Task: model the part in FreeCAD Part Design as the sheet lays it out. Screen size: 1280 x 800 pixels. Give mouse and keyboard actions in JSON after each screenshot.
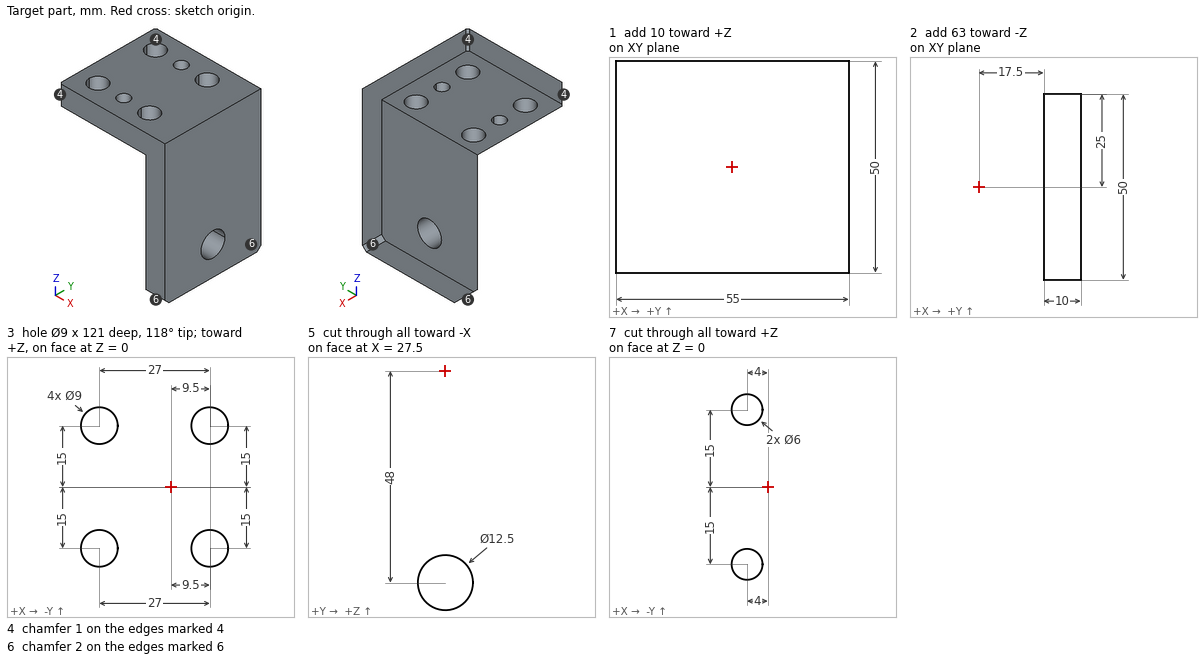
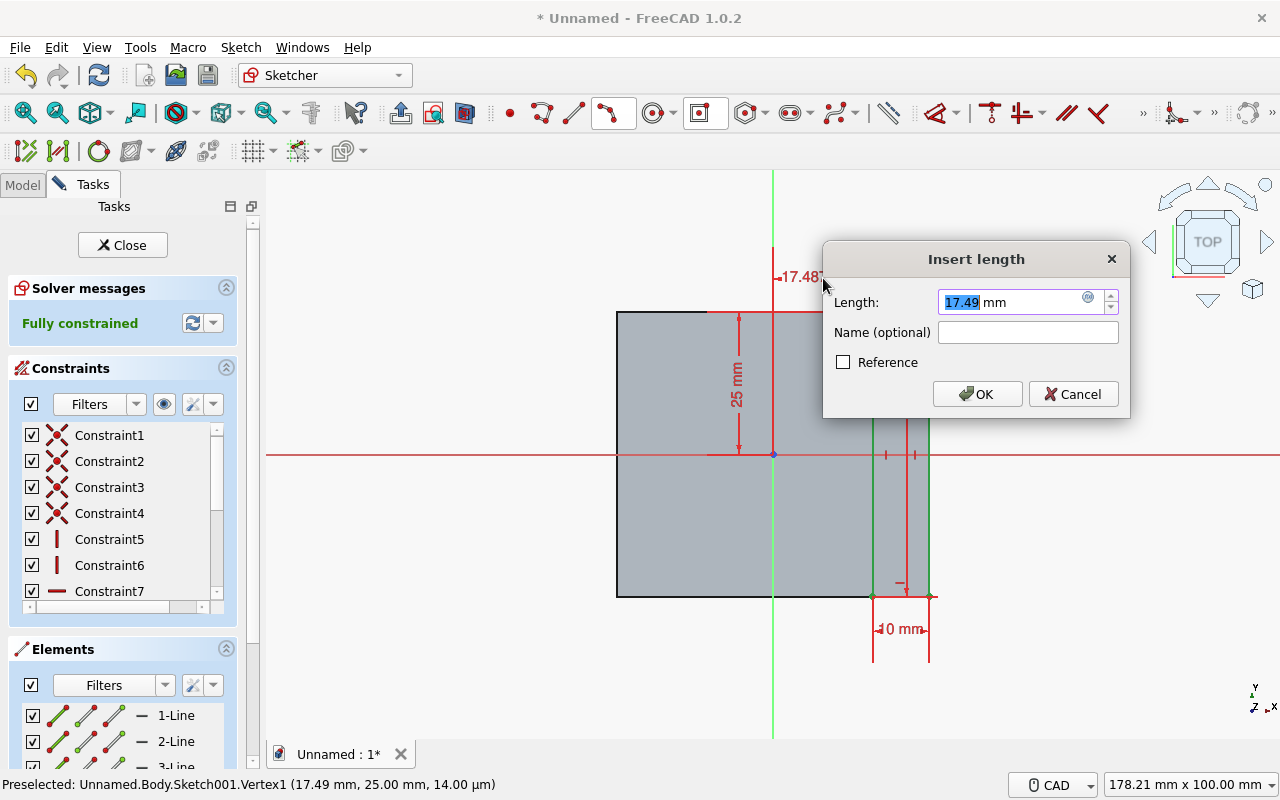
{"action": "type", "text": "17.5"}
{"action": "key", "text": "Return"}
{"action": "key", "text": "Escape"}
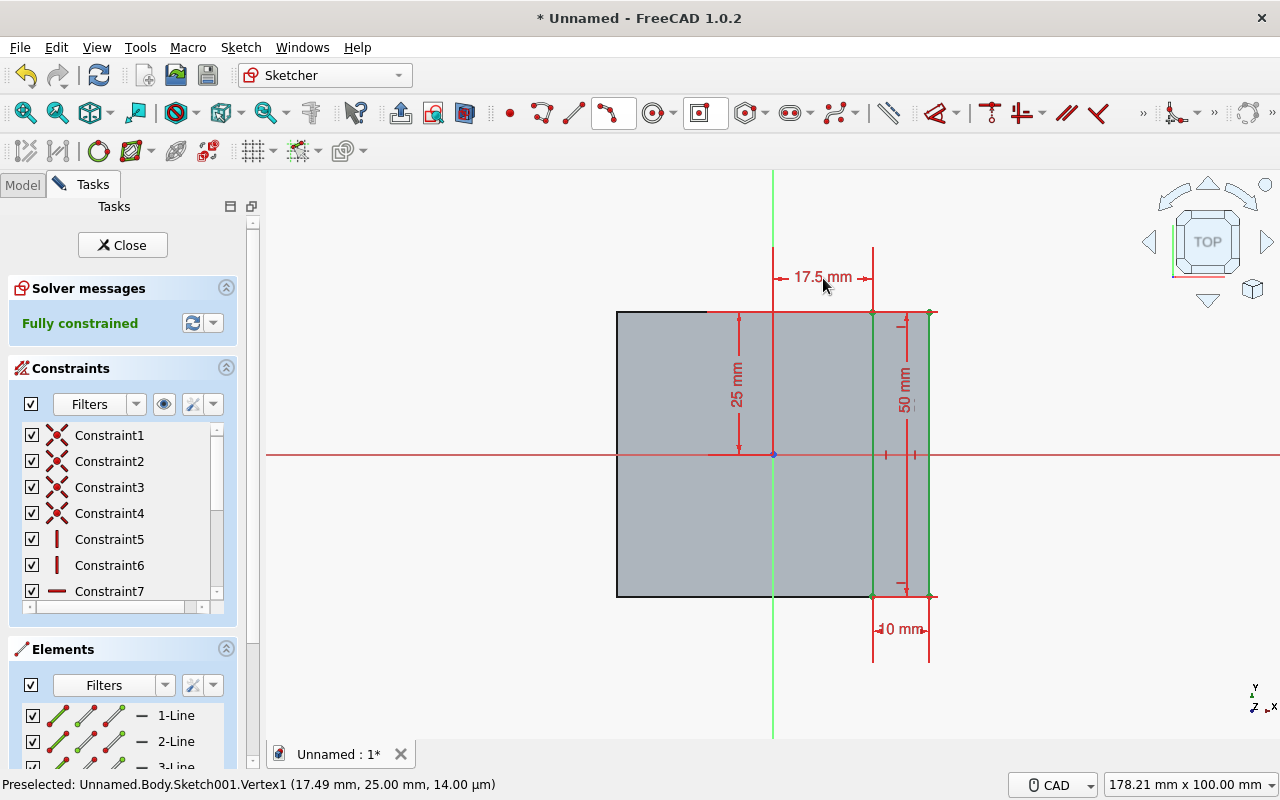
{"action": "left_click", "coordinate": [123, 245]}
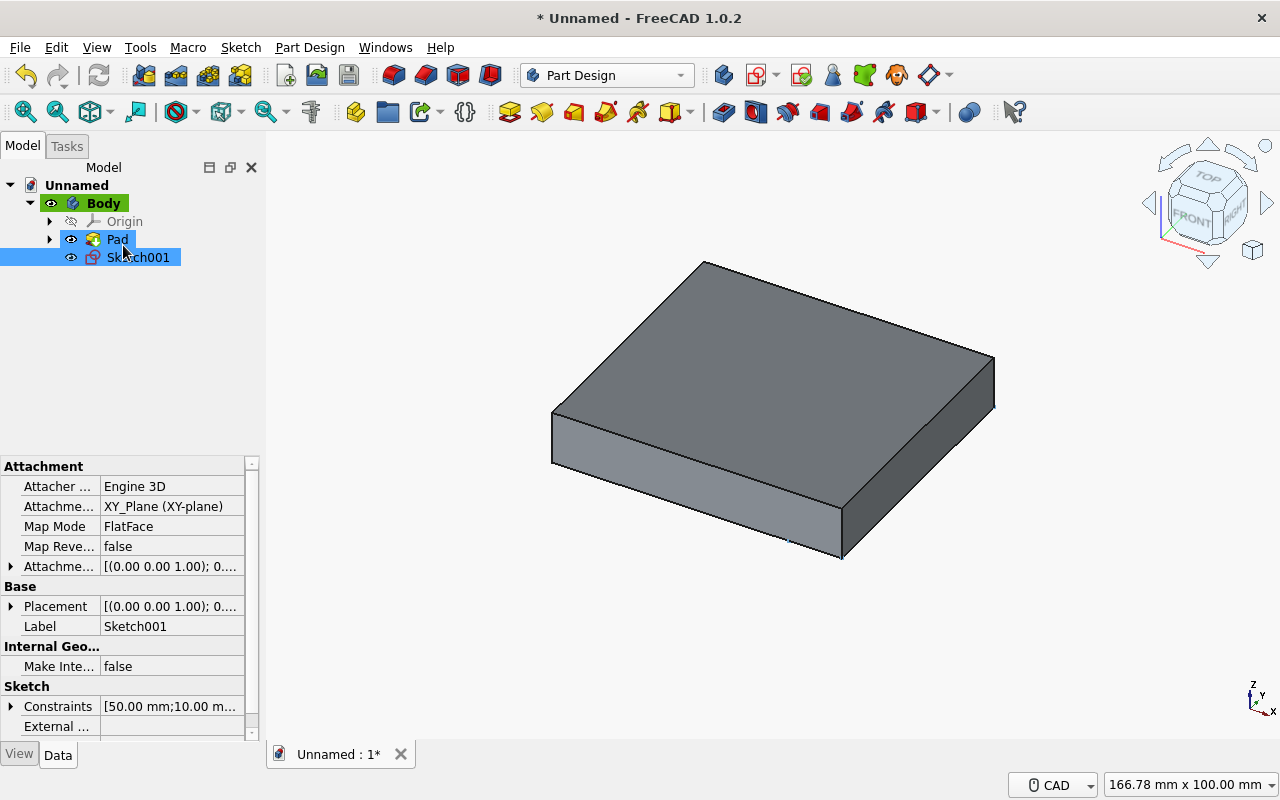
{"action": "left_click", "coordinate": [510, 112]}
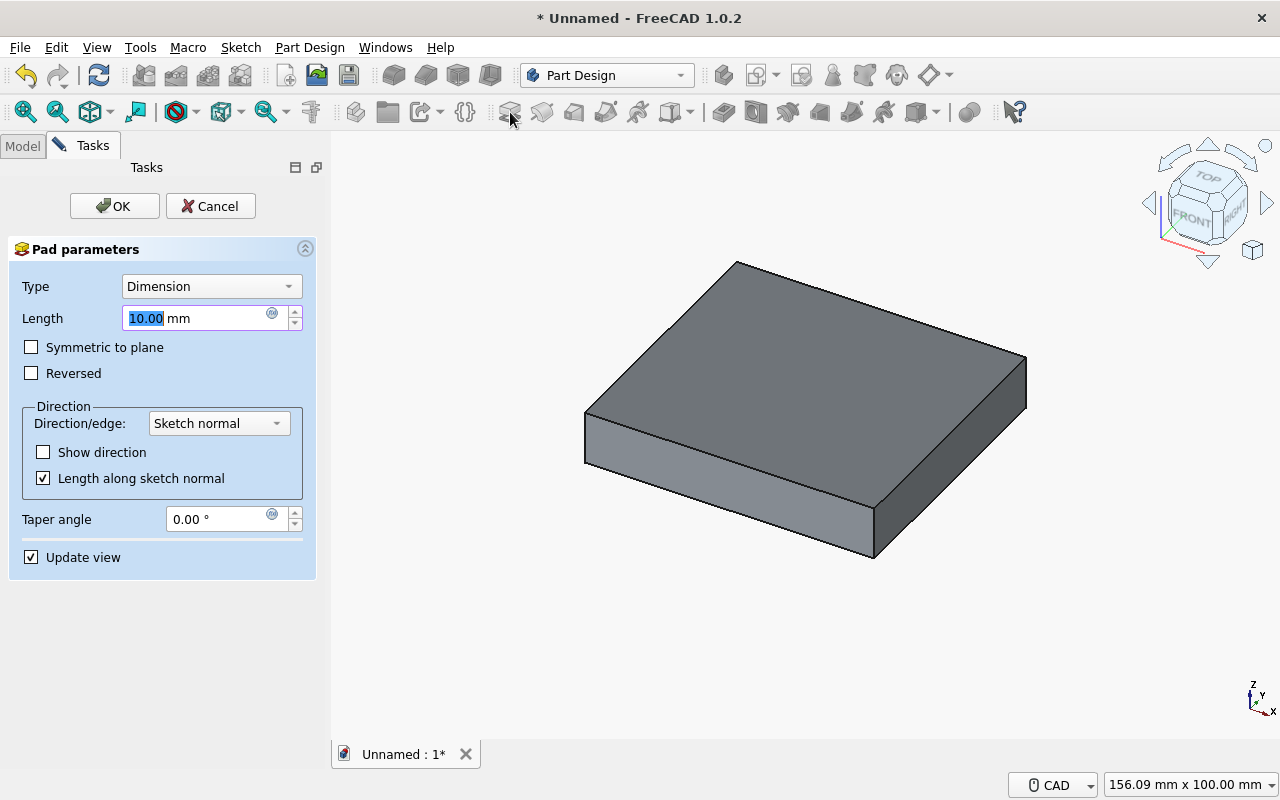
{"action": "type", "text": "63"}
{"action": "key", "text": "Tab"}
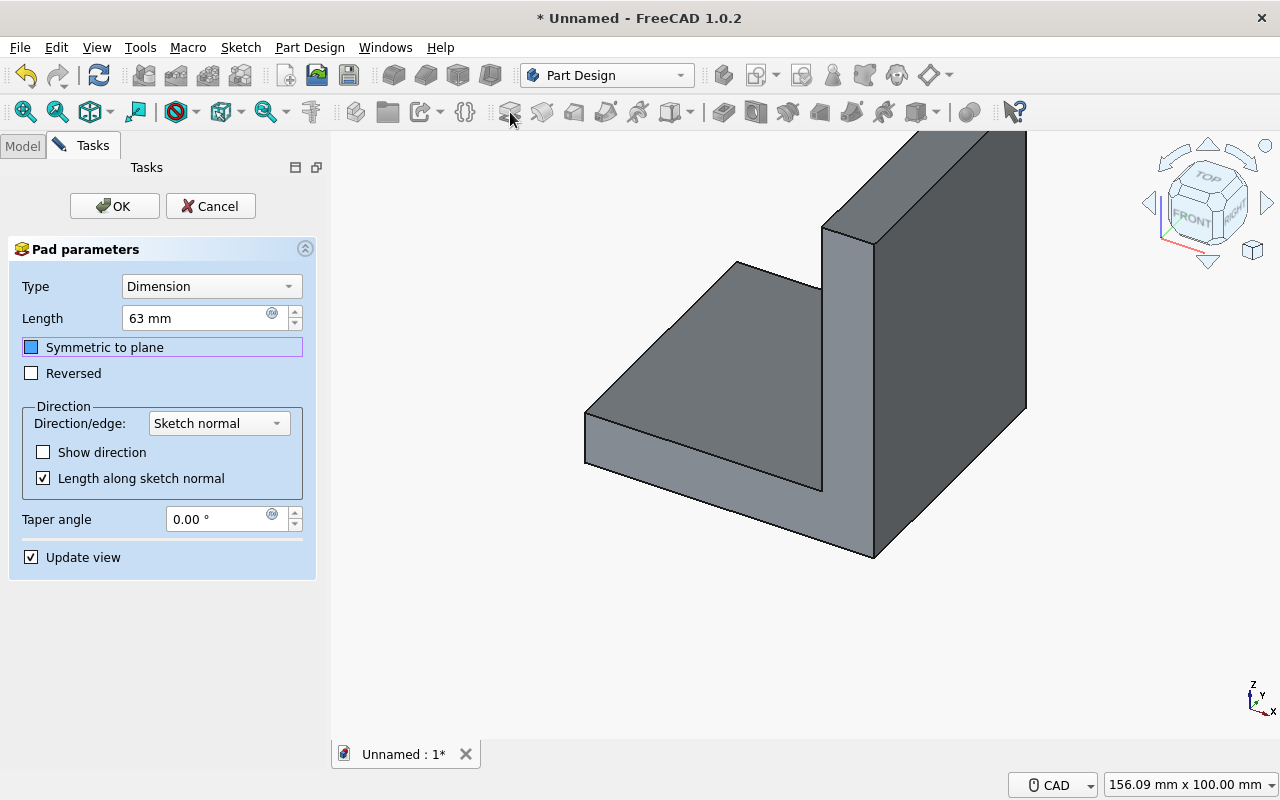
{"action": "left_click", "coordinate": [30, 373]}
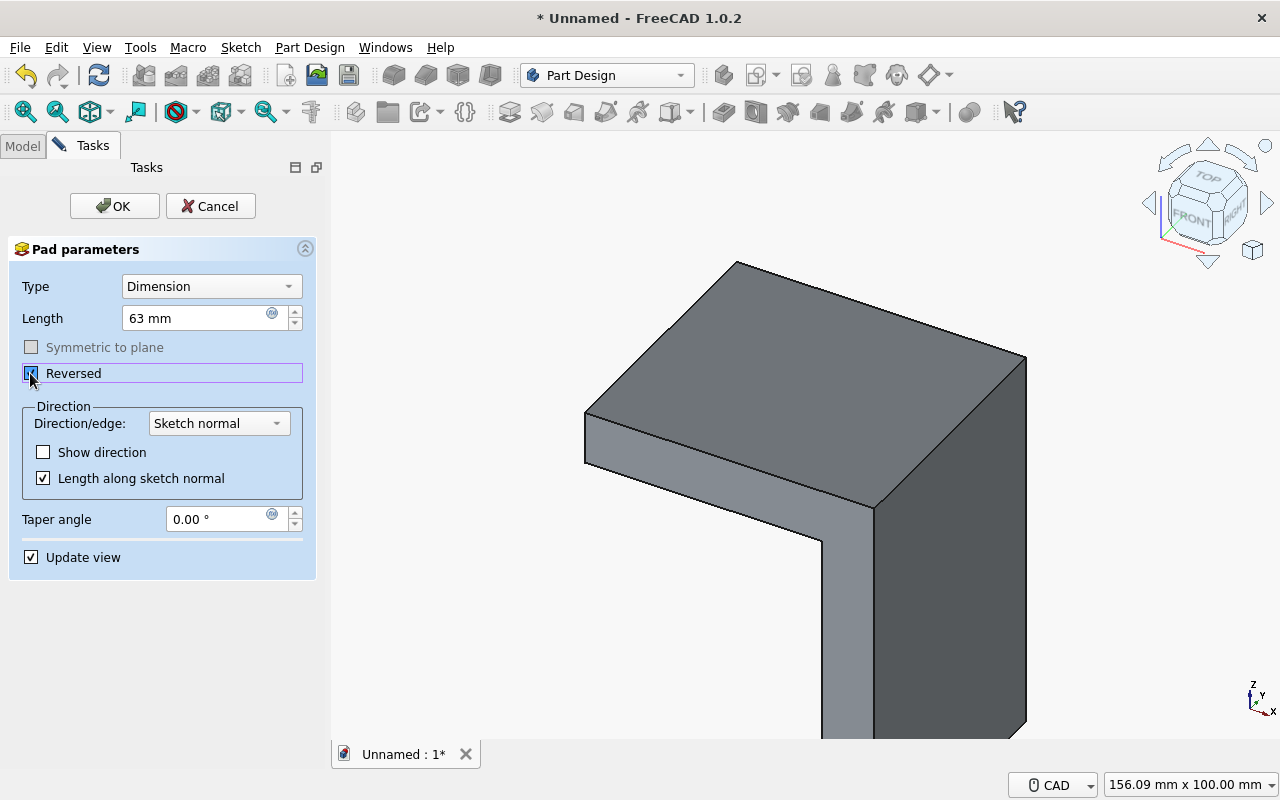
{"action": "left_click", "coordinate": [115, 206]}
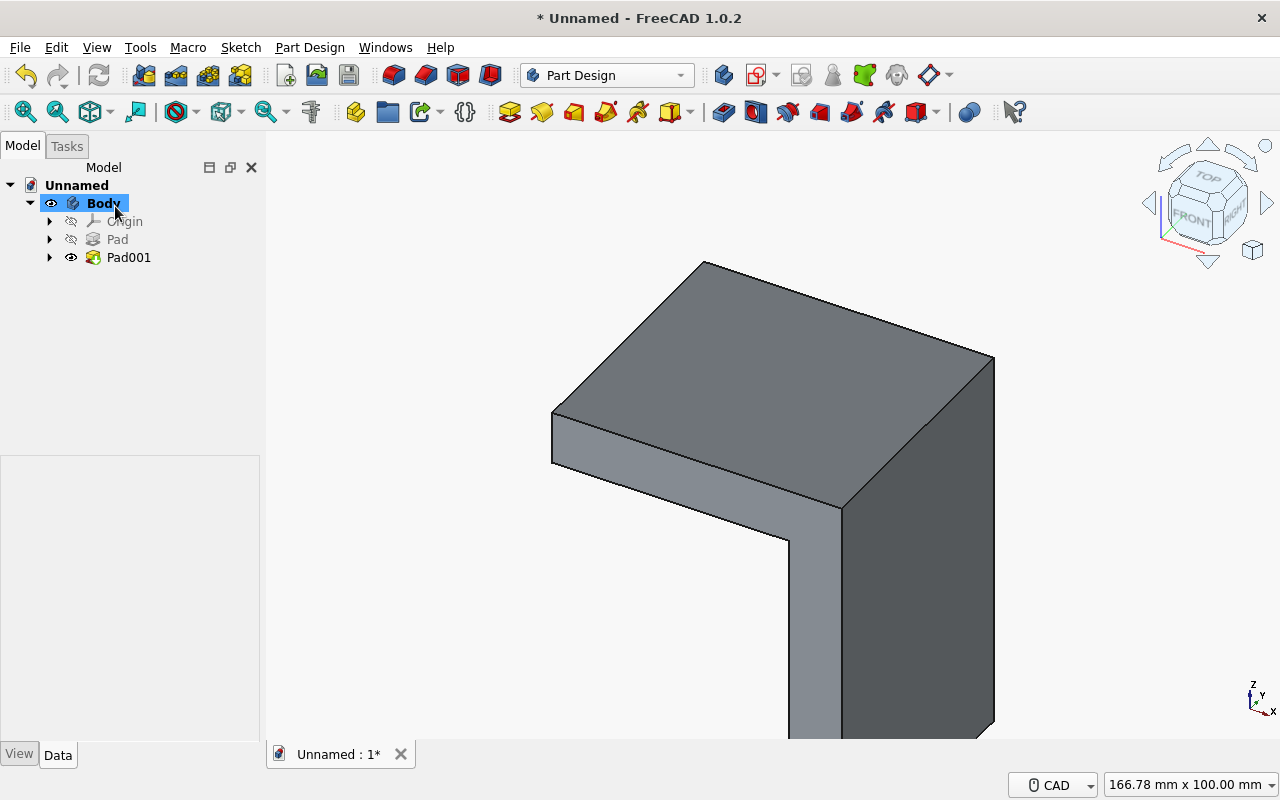
{"action": "key", "text": "v f"}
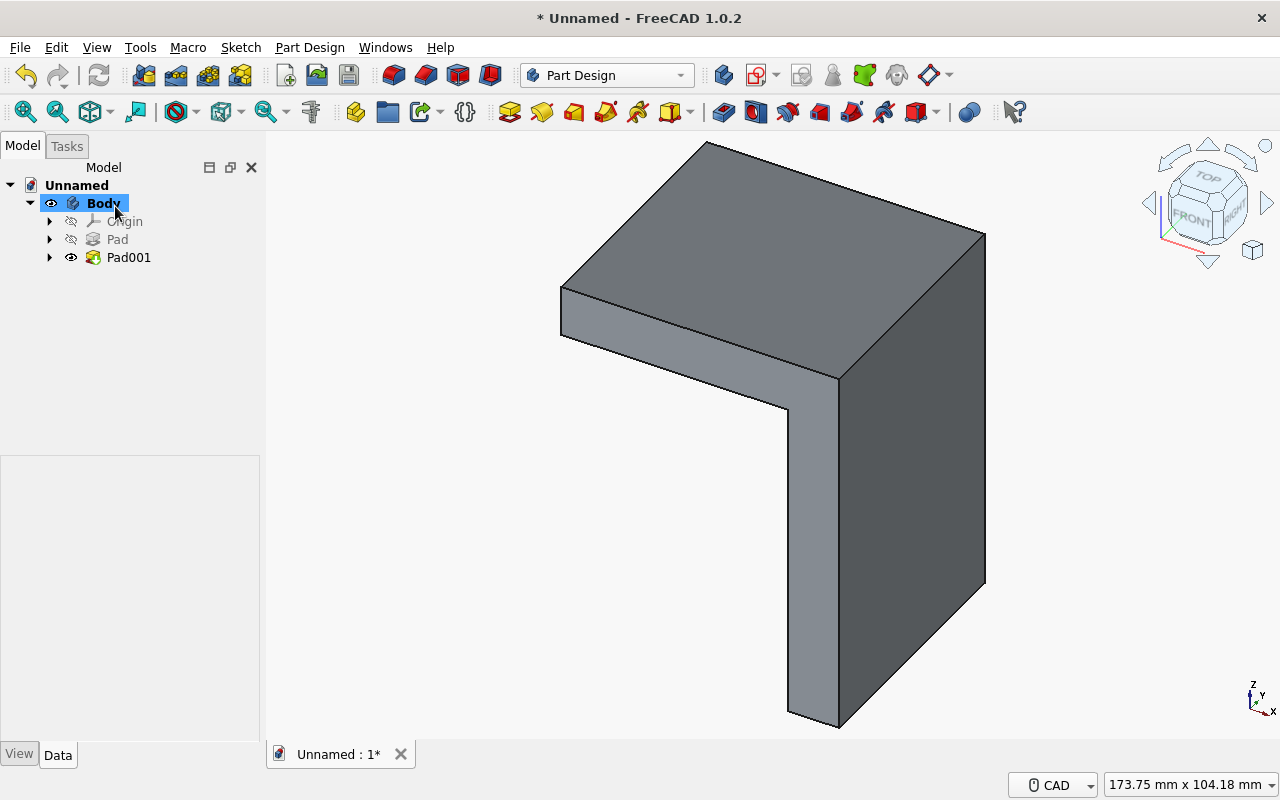
{"action": "key", "text": "5"}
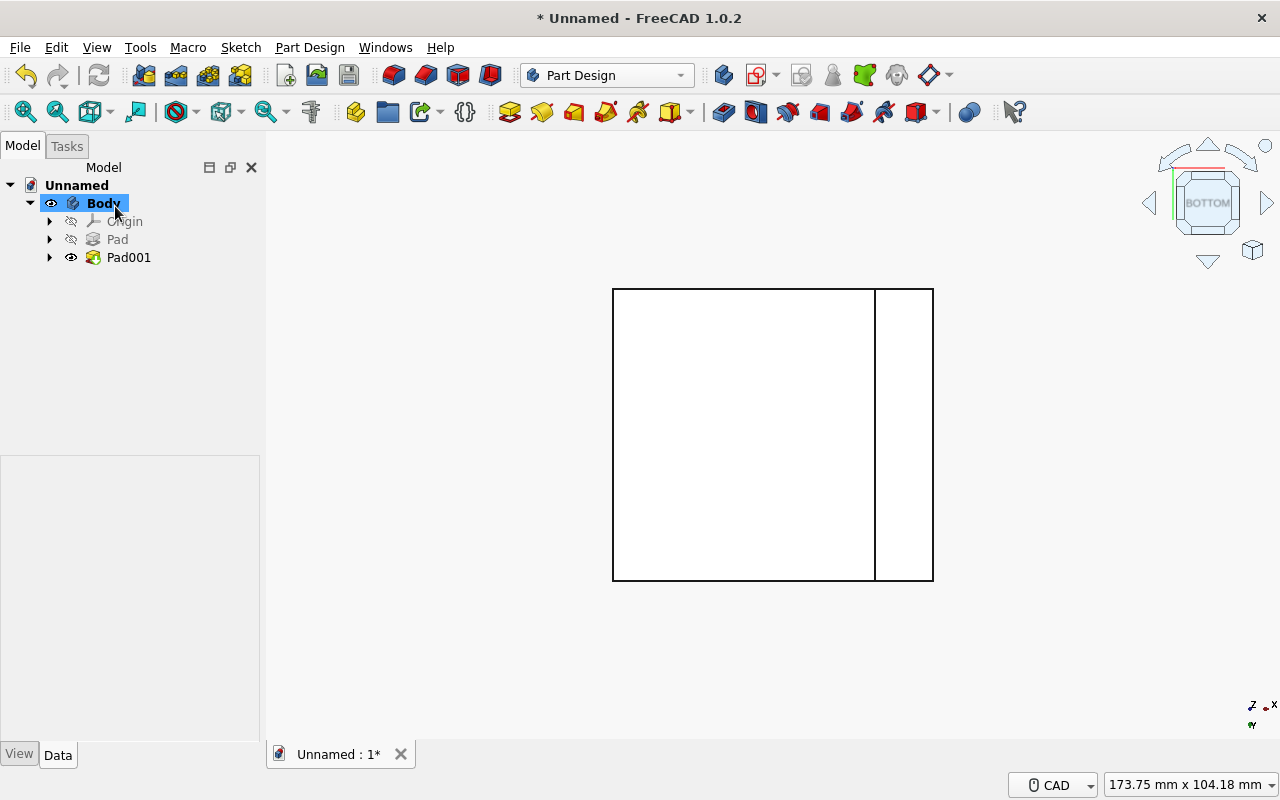
{"action": "left_click", "coordinate": [744, 434]}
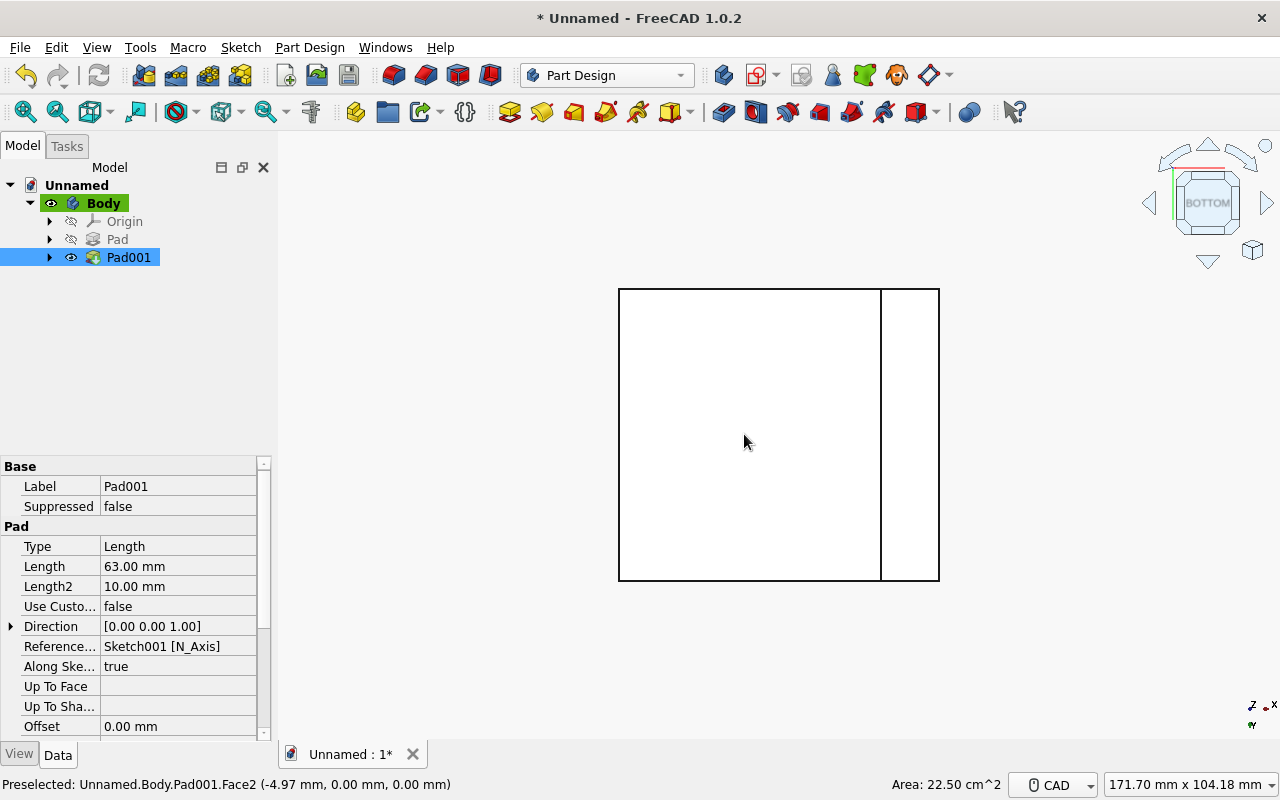
{"action": "left_click", "coordinate": [756, 76]}